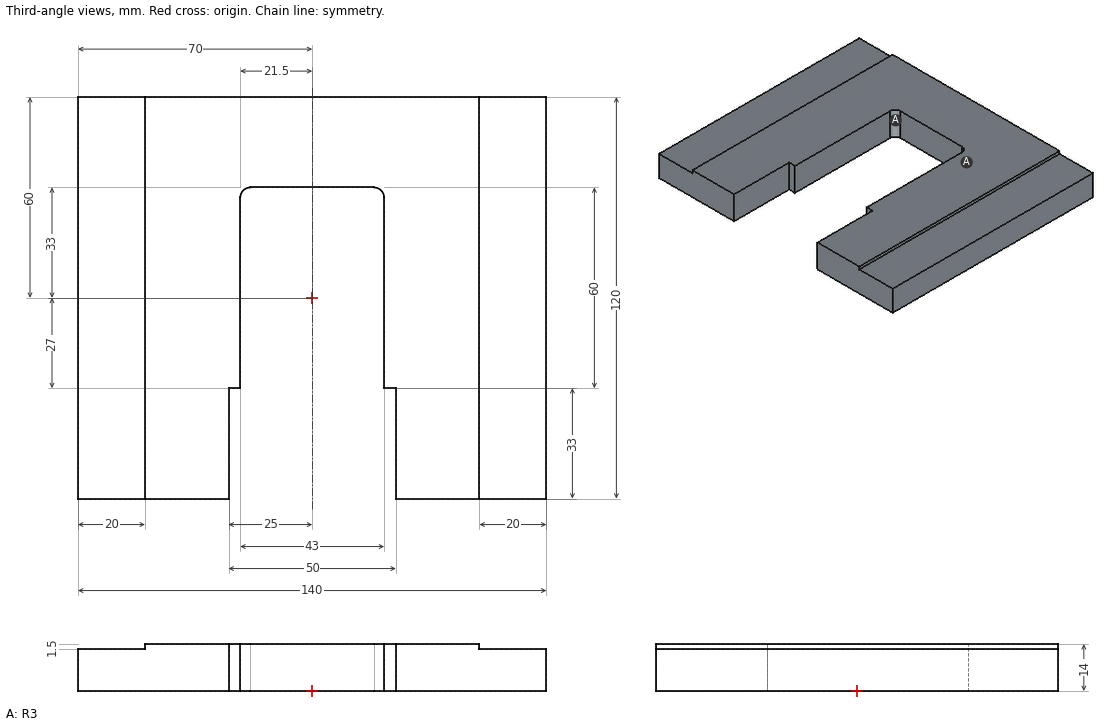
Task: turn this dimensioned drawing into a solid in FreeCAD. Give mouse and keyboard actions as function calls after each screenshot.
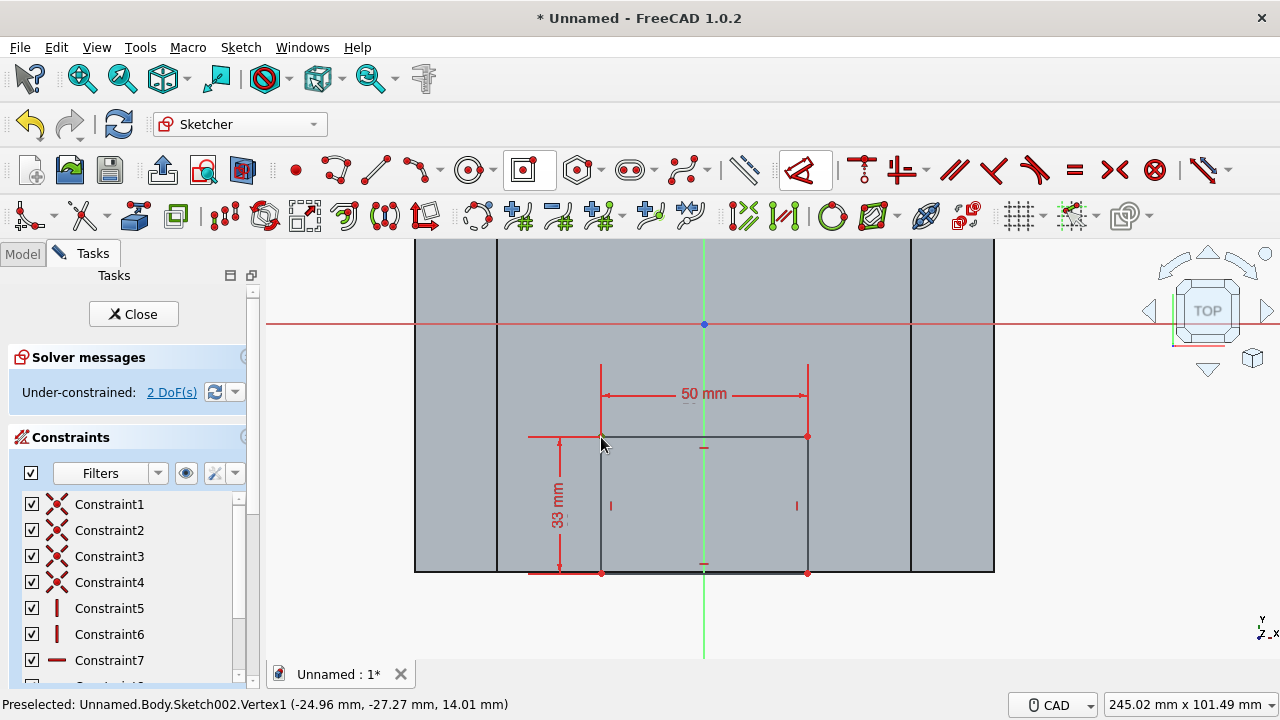
click(826, 170)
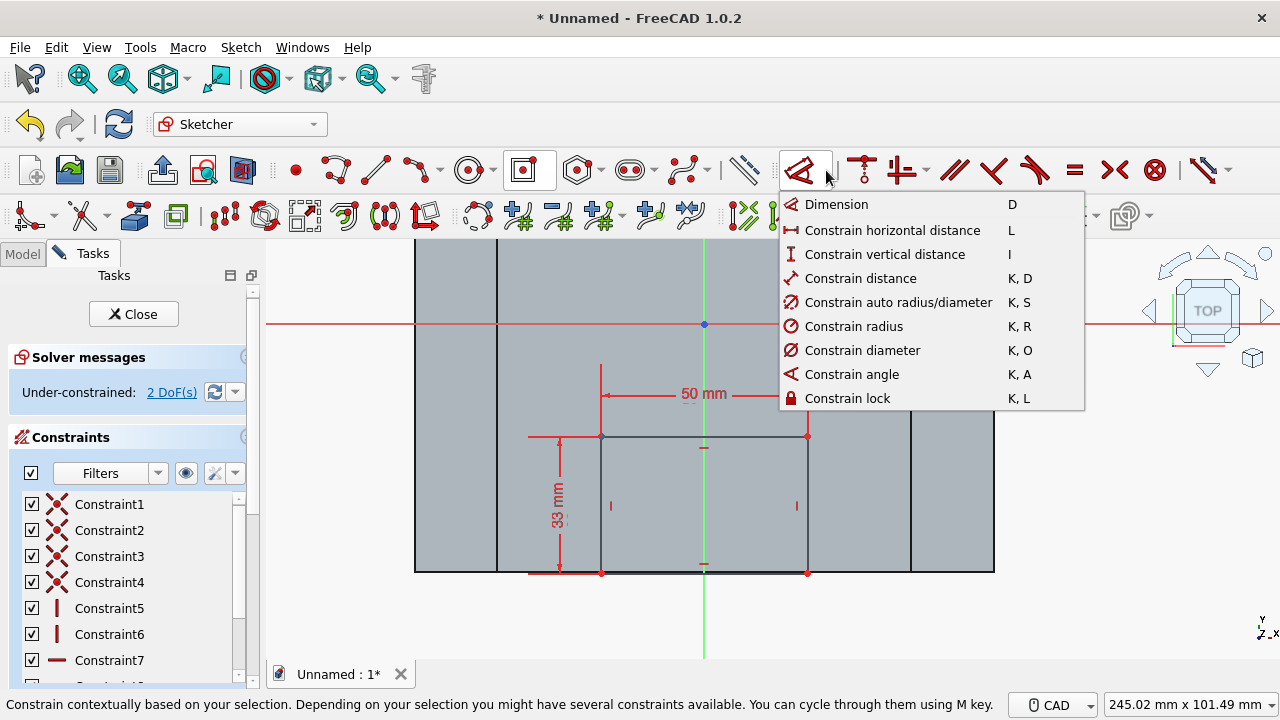
click(932, 230)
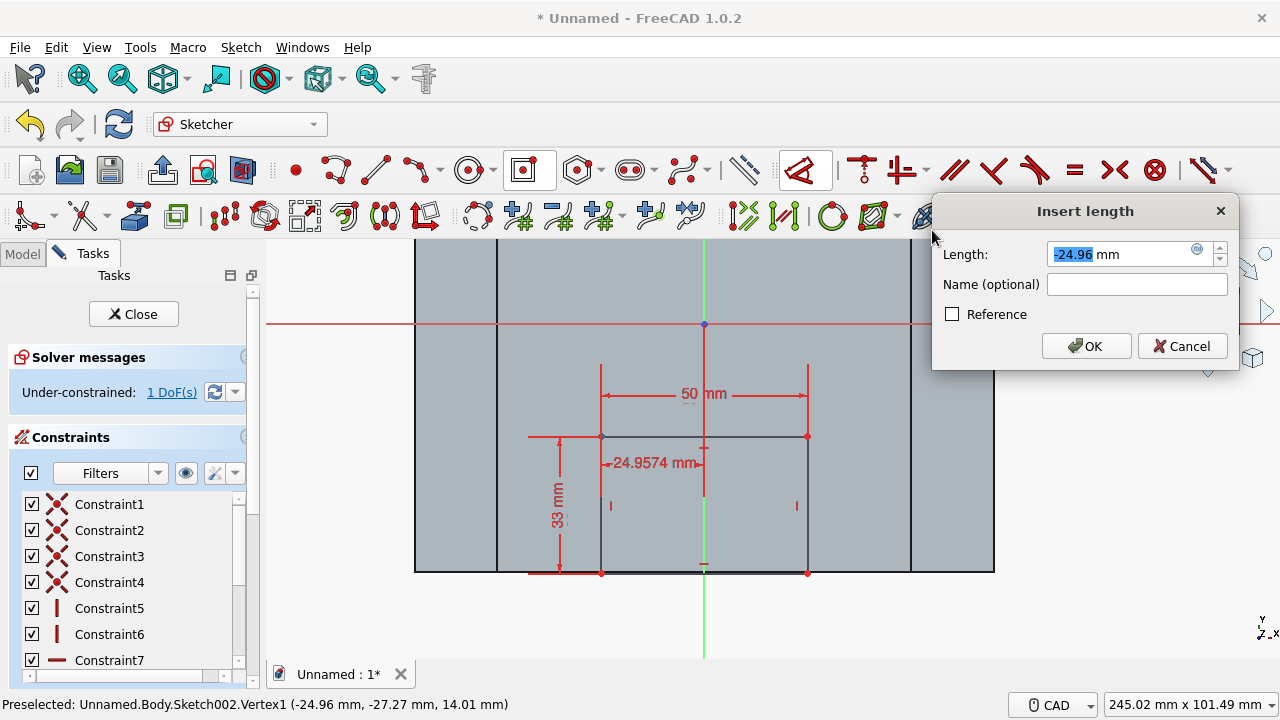
text(-25)
key(Return)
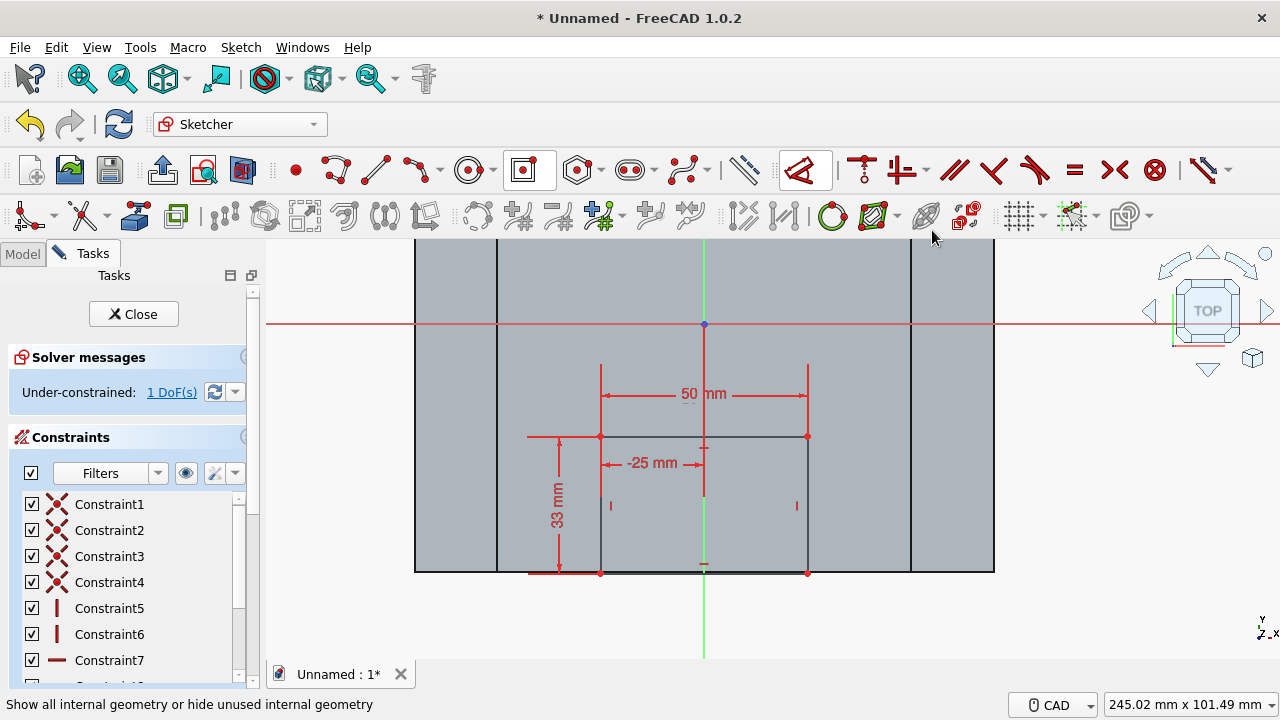
click(601, 437)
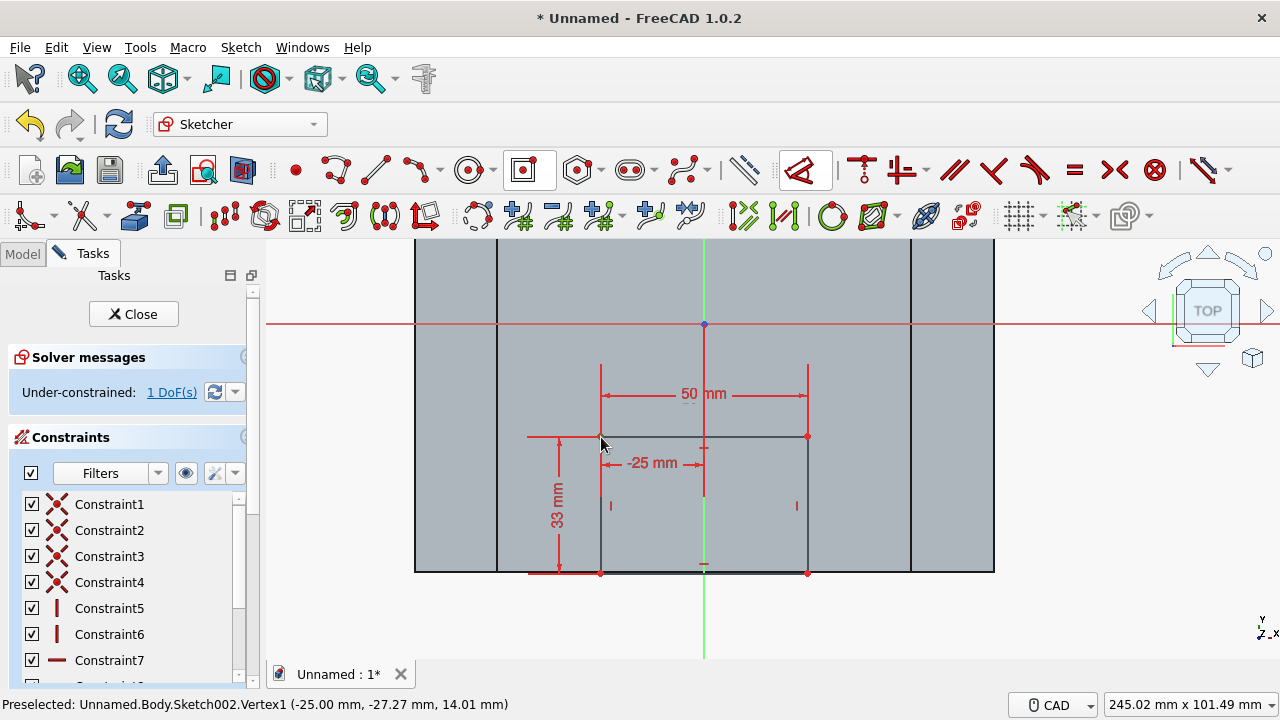
click(826, 170)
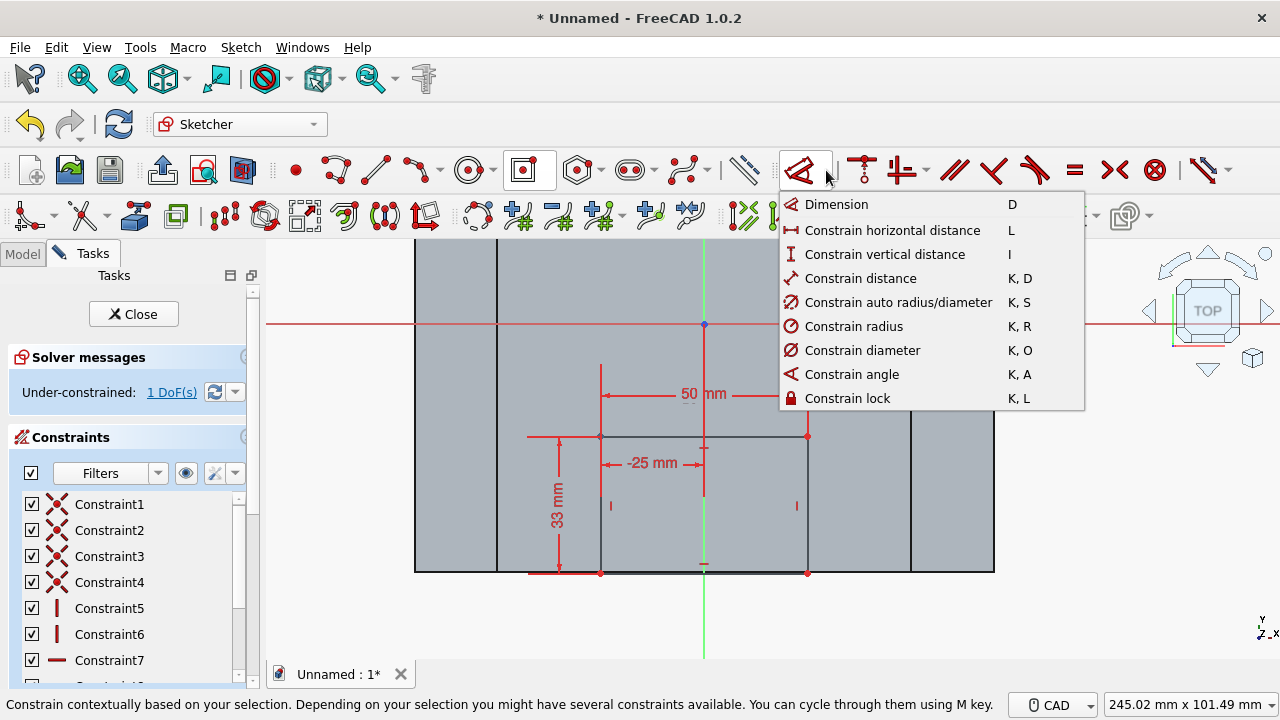
click(932, 254)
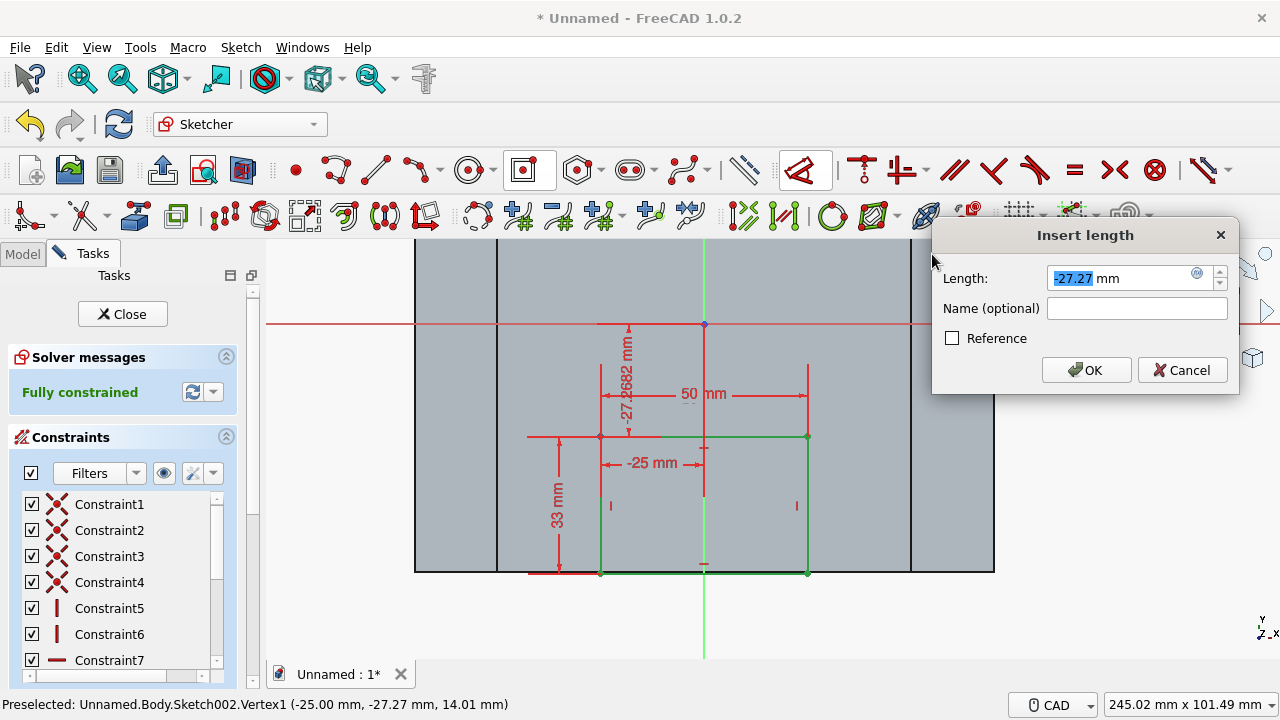
text(-27)
key(Return)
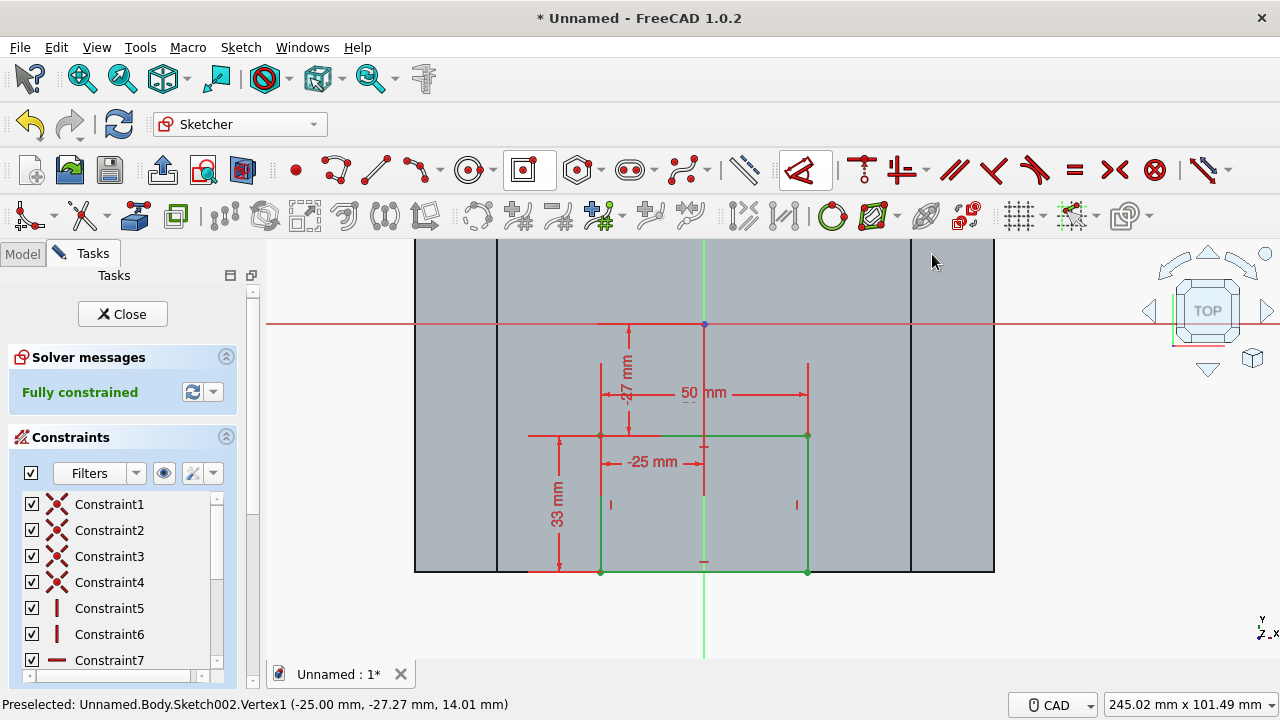
click(123, 314)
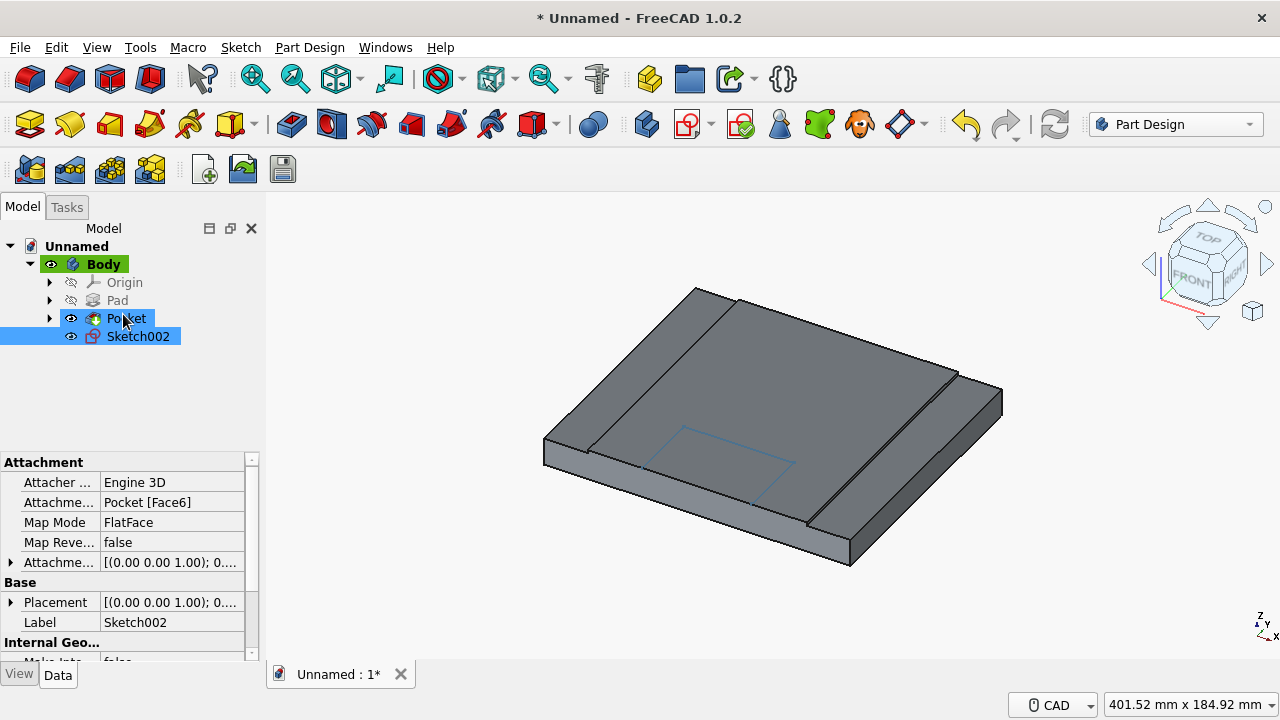
click(292, 124)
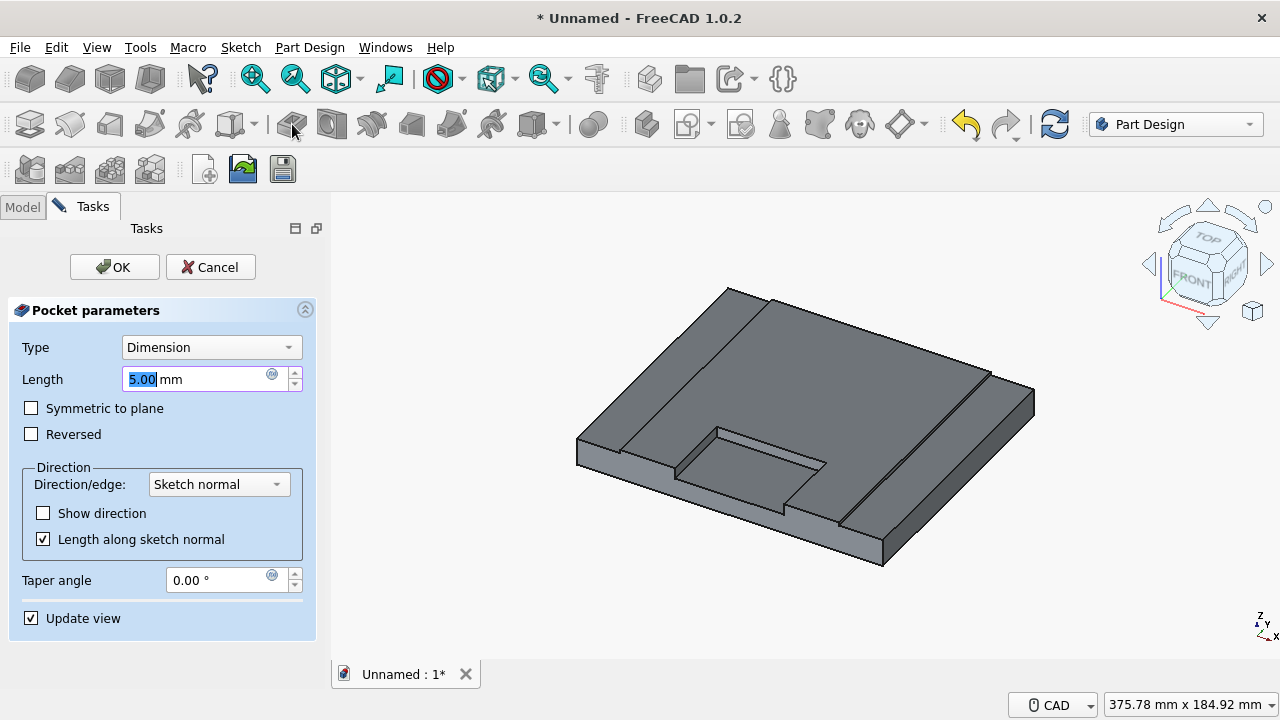
click(212, 348)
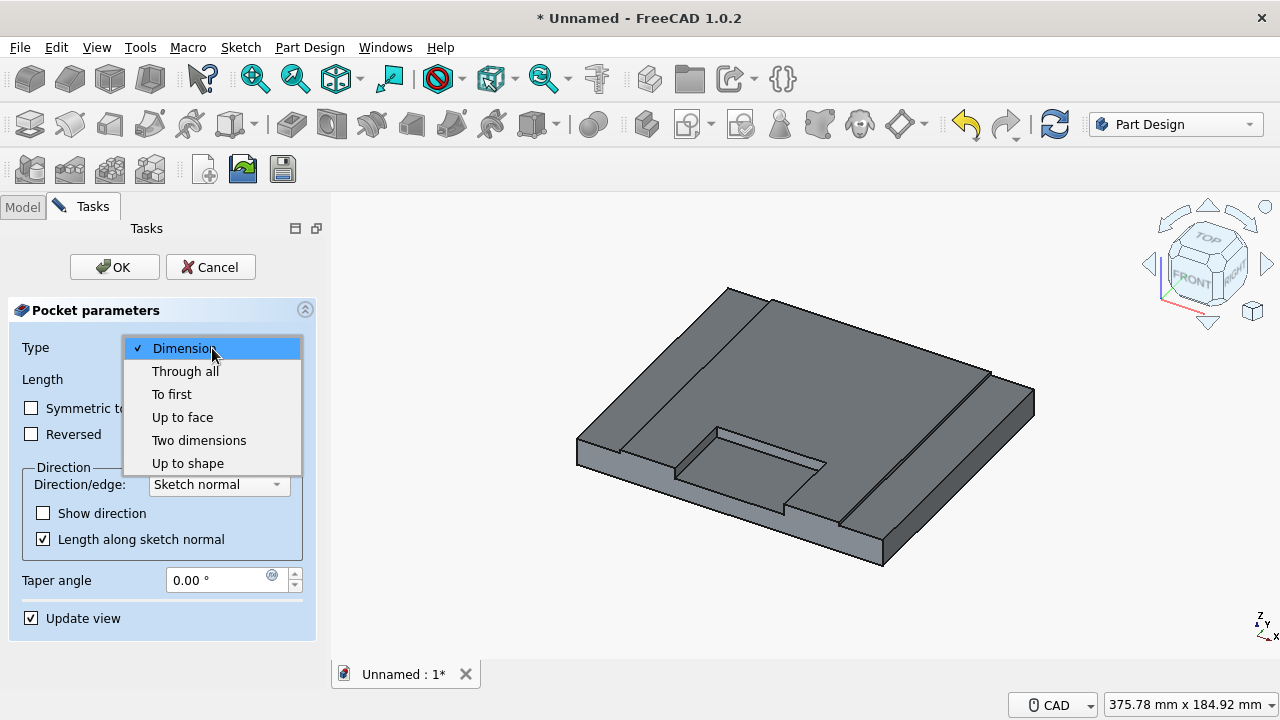
click(212, 394)